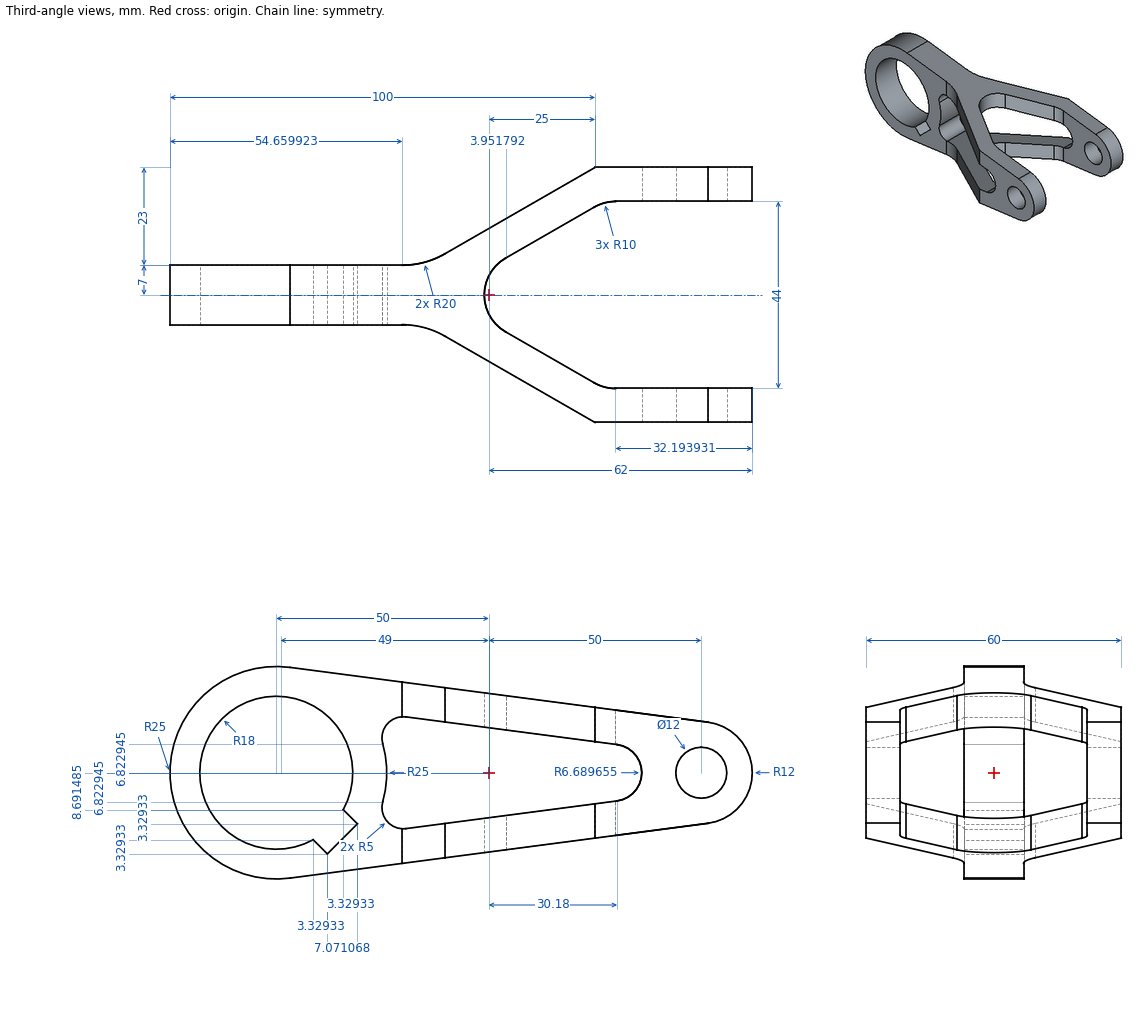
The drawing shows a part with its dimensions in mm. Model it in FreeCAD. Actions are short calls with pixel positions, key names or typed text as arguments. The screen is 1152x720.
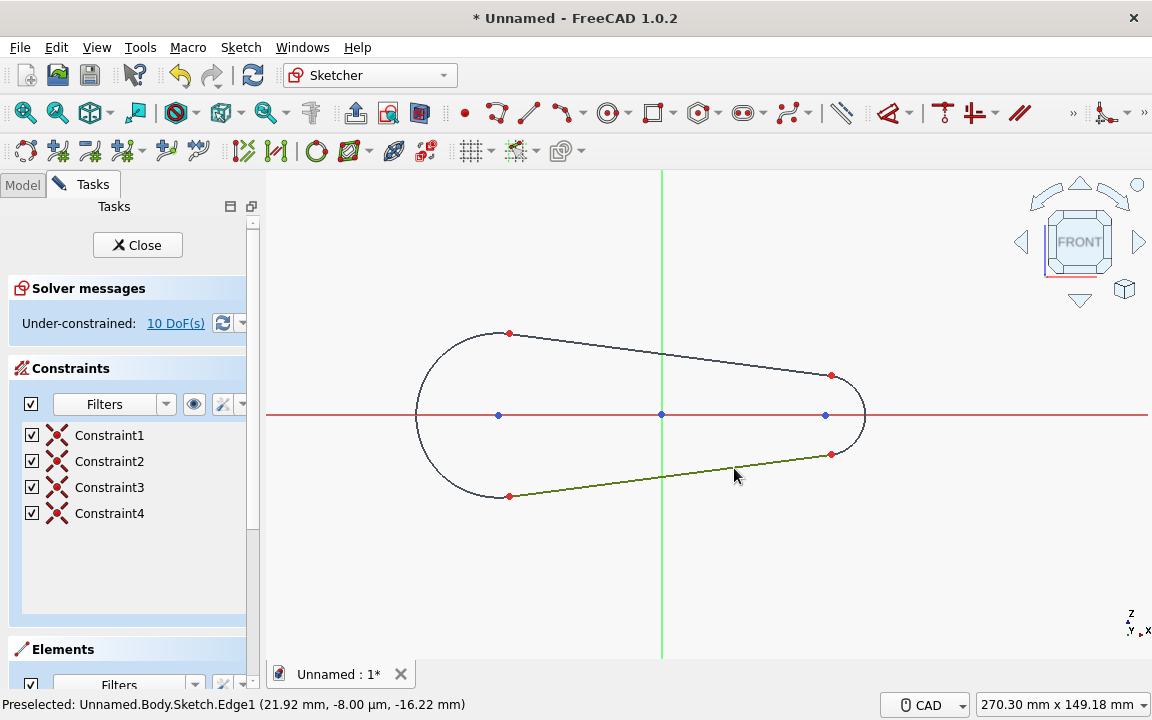
click(435, 364)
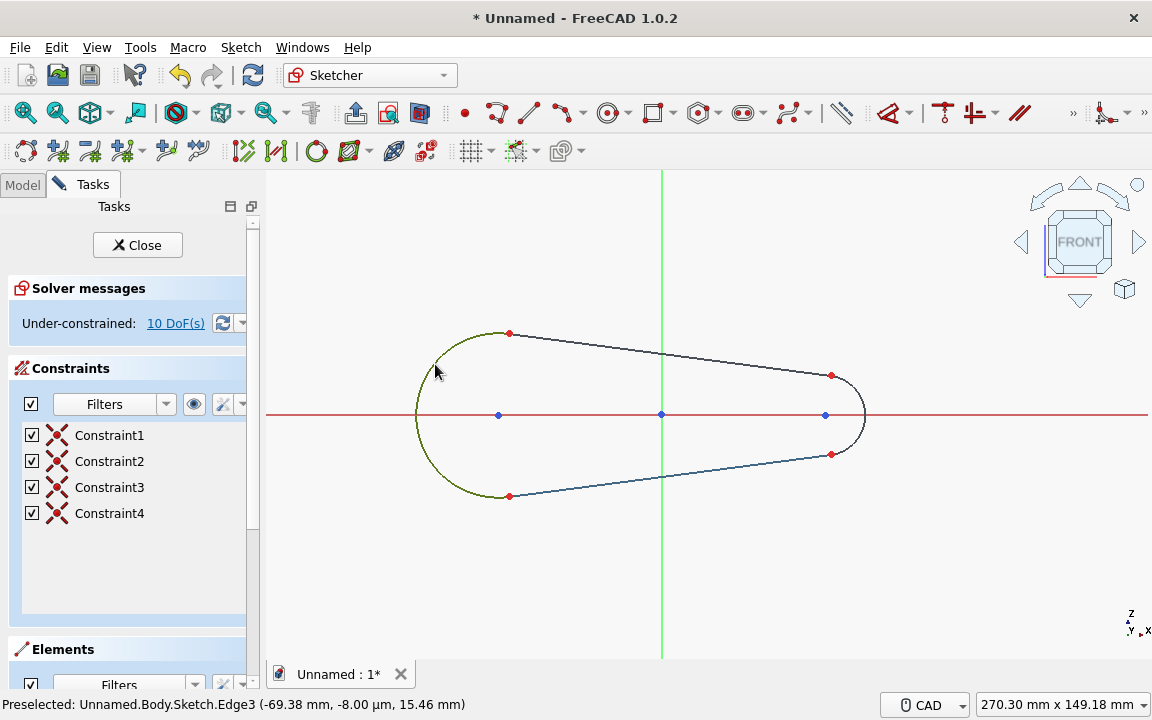
key(t)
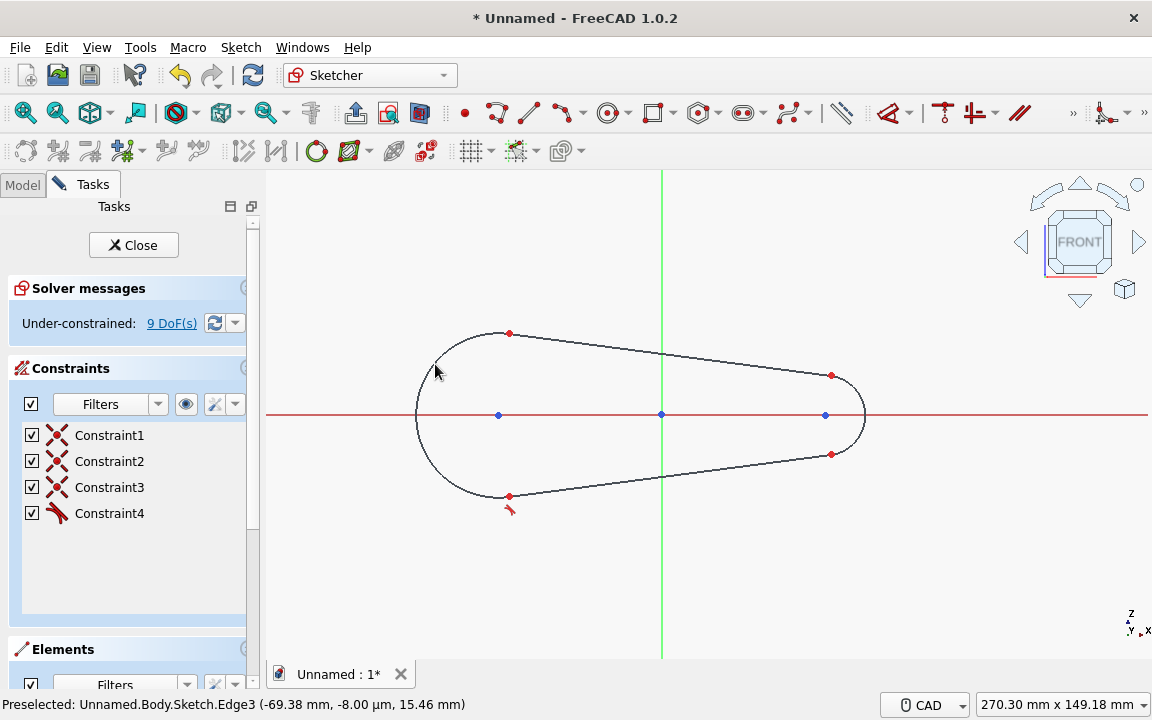
click(734, 468)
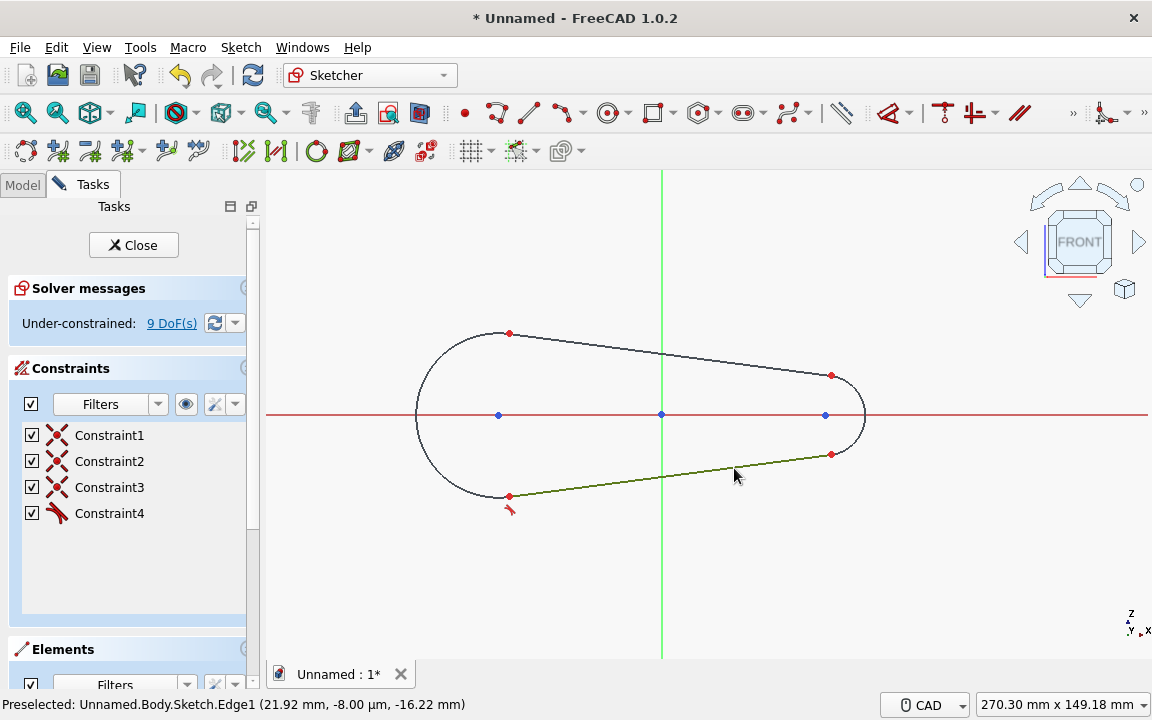
click(859, 437)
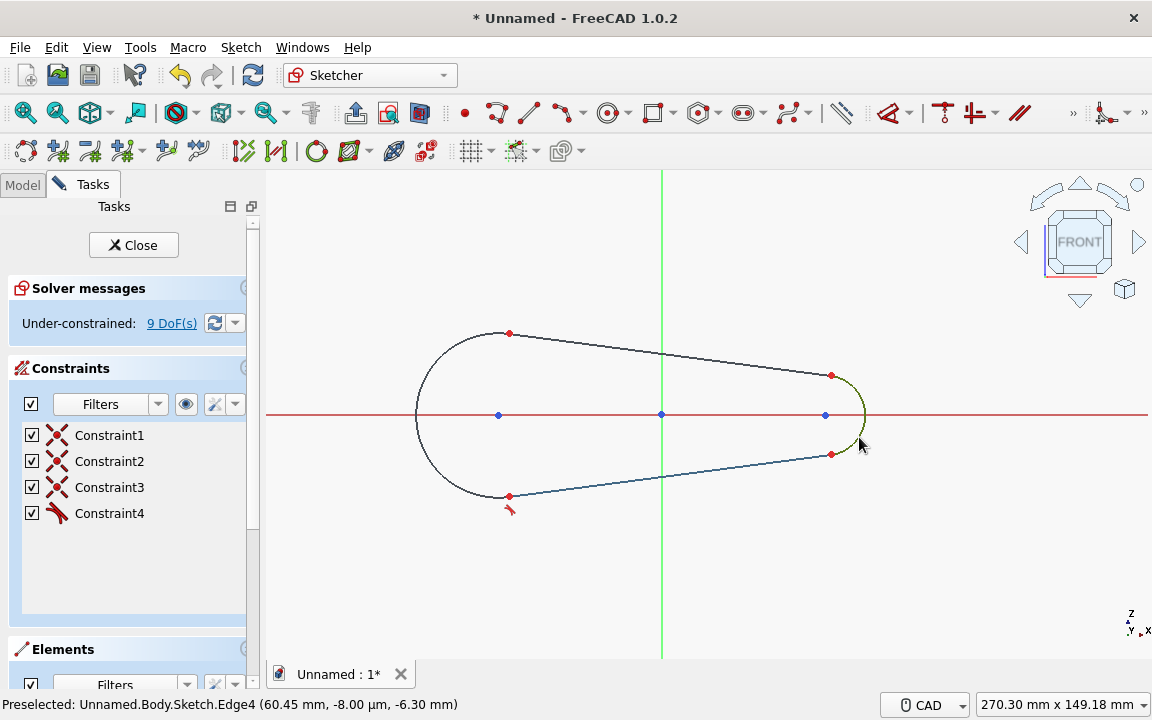
key(t)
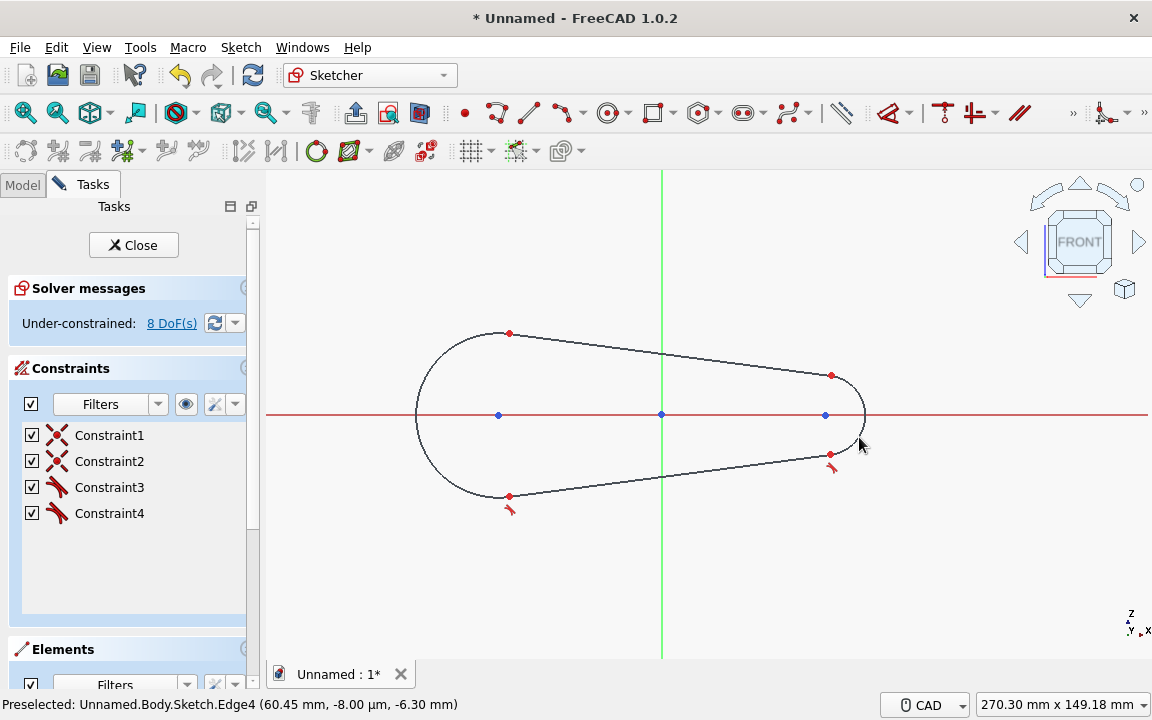
click(606, 347)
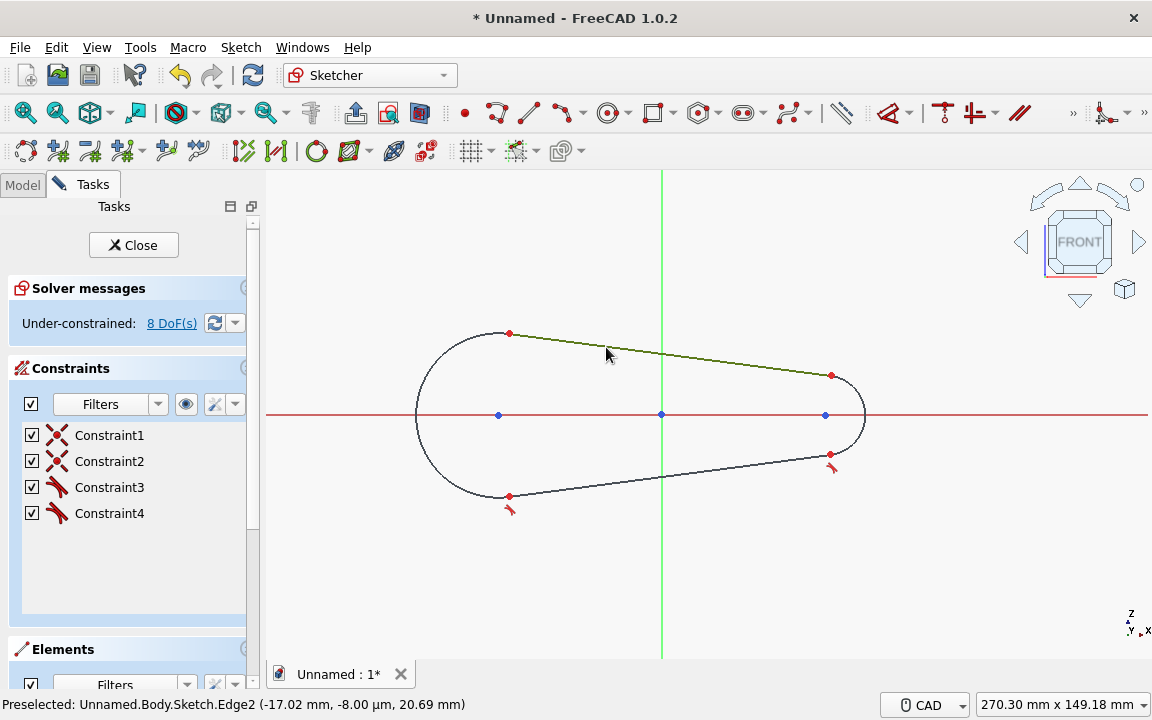
click(434, 364)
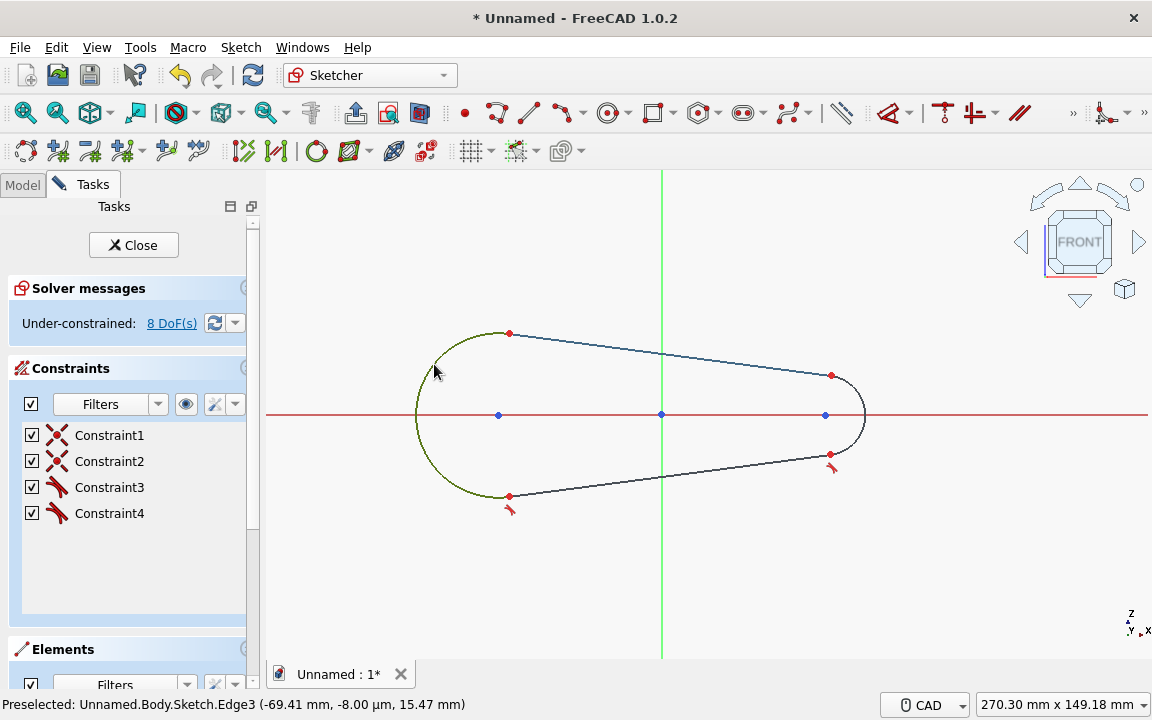
key(t)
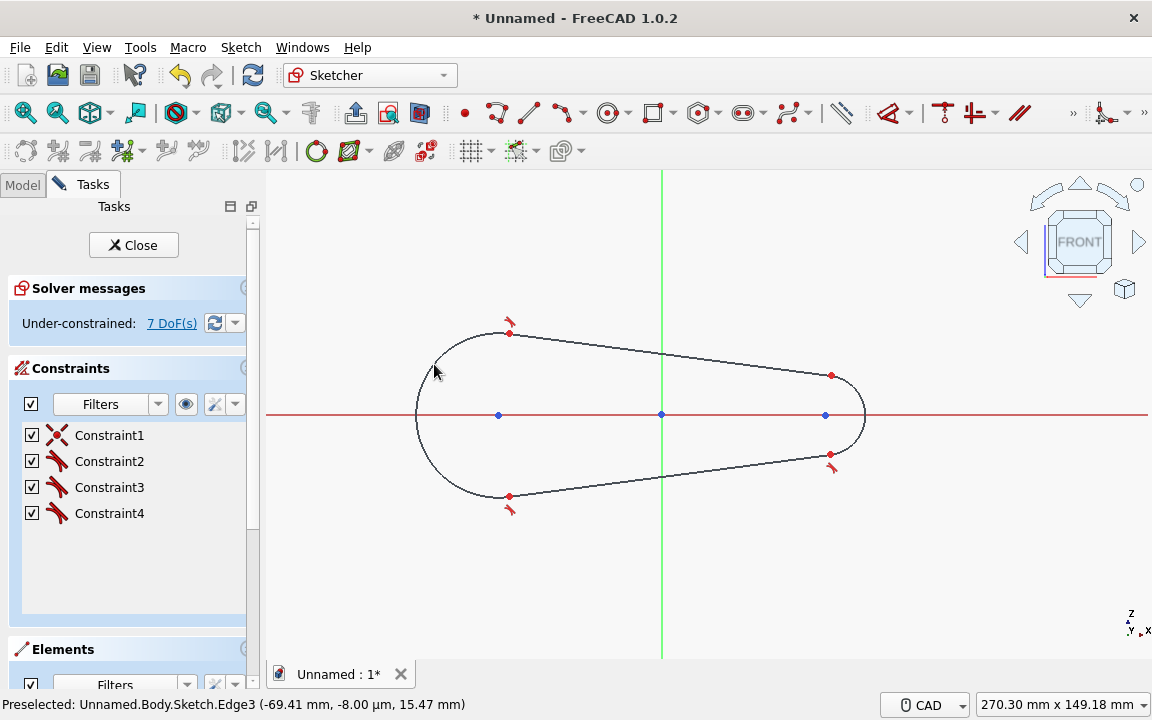
click(606, 347)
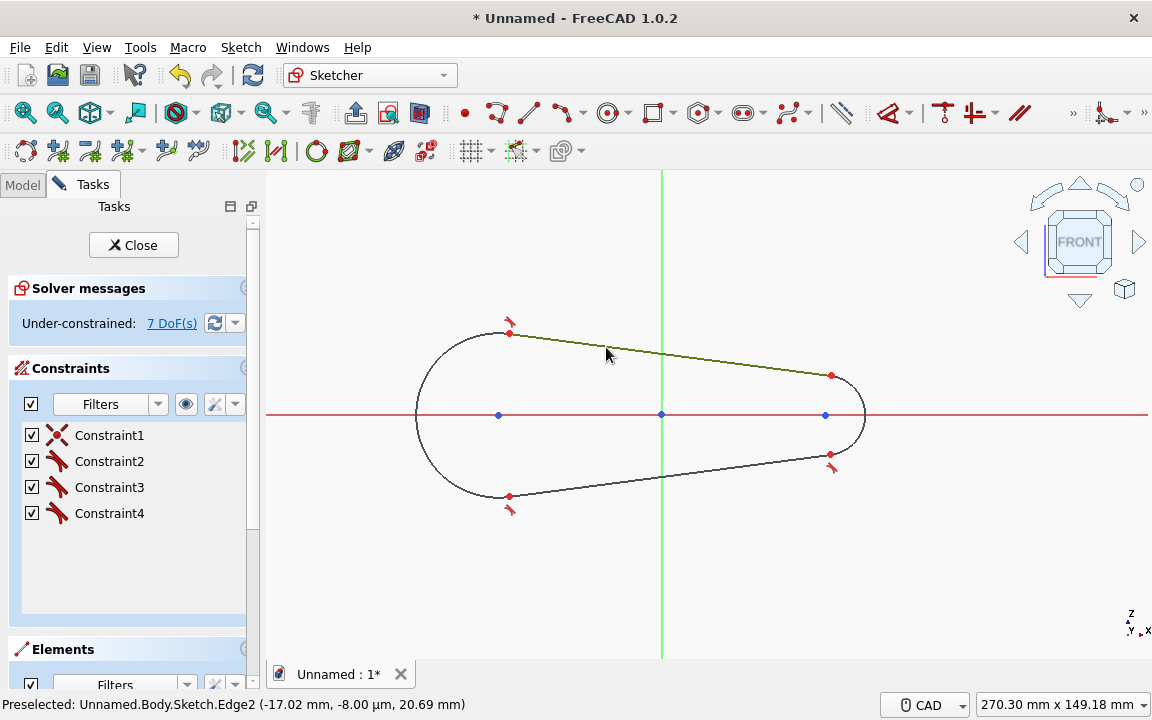
click(859, 437)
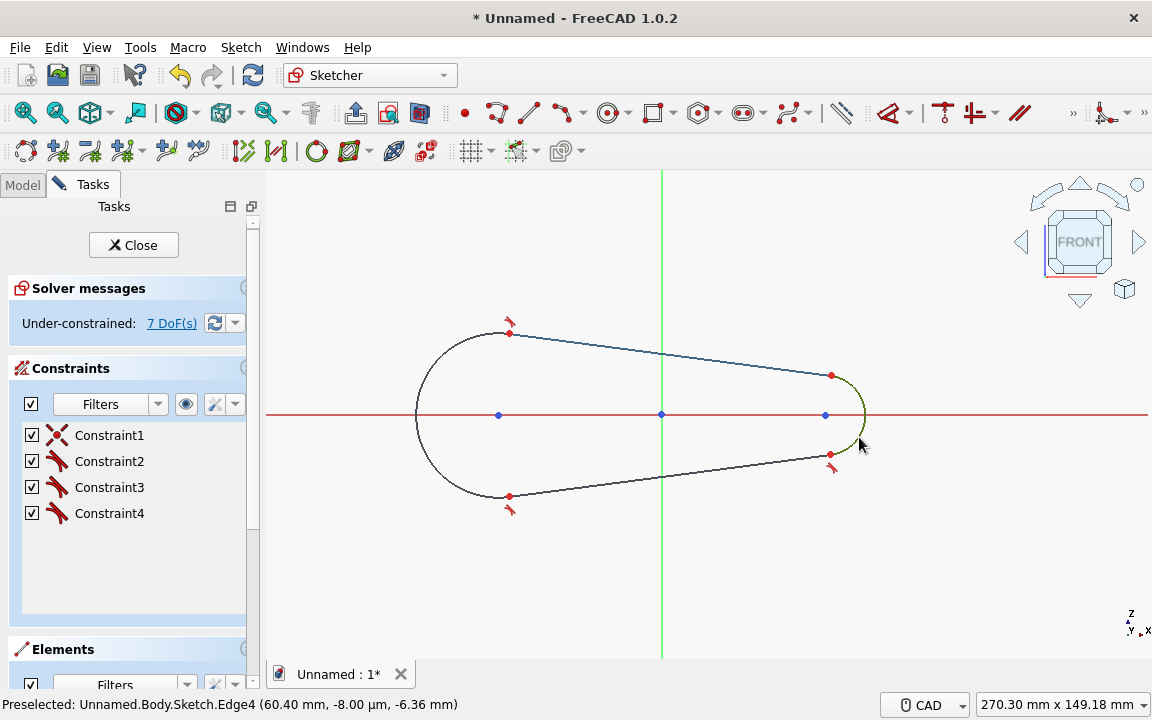
key(t)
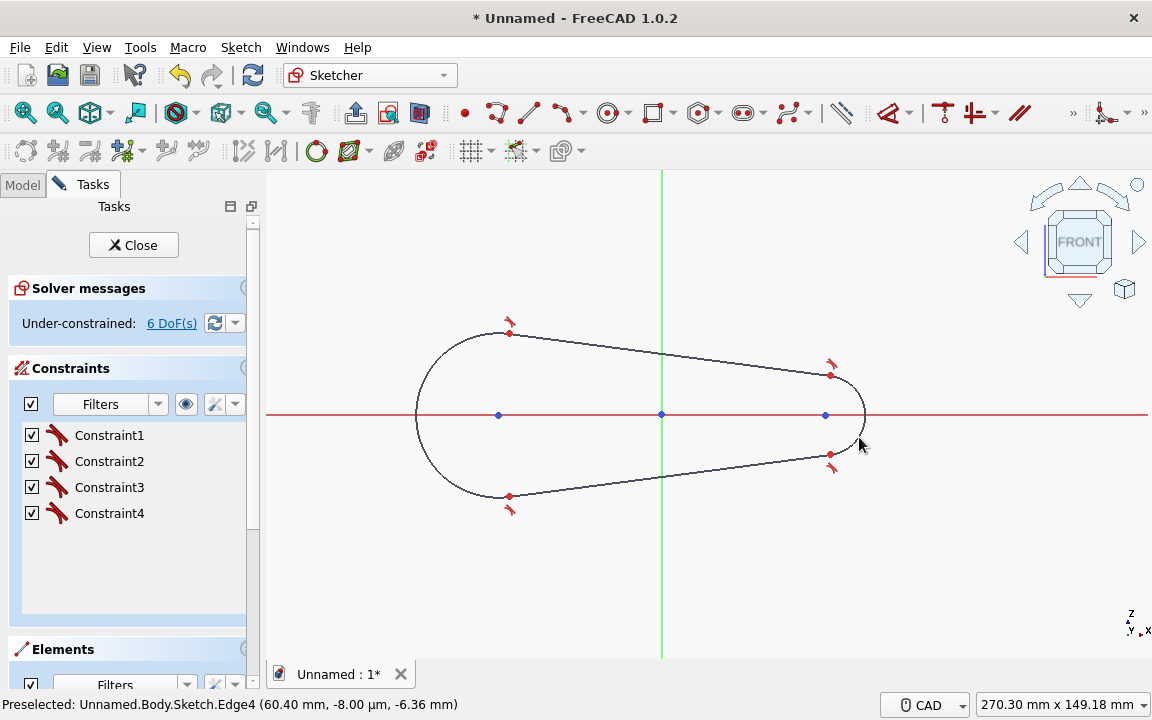
click(498, 416)